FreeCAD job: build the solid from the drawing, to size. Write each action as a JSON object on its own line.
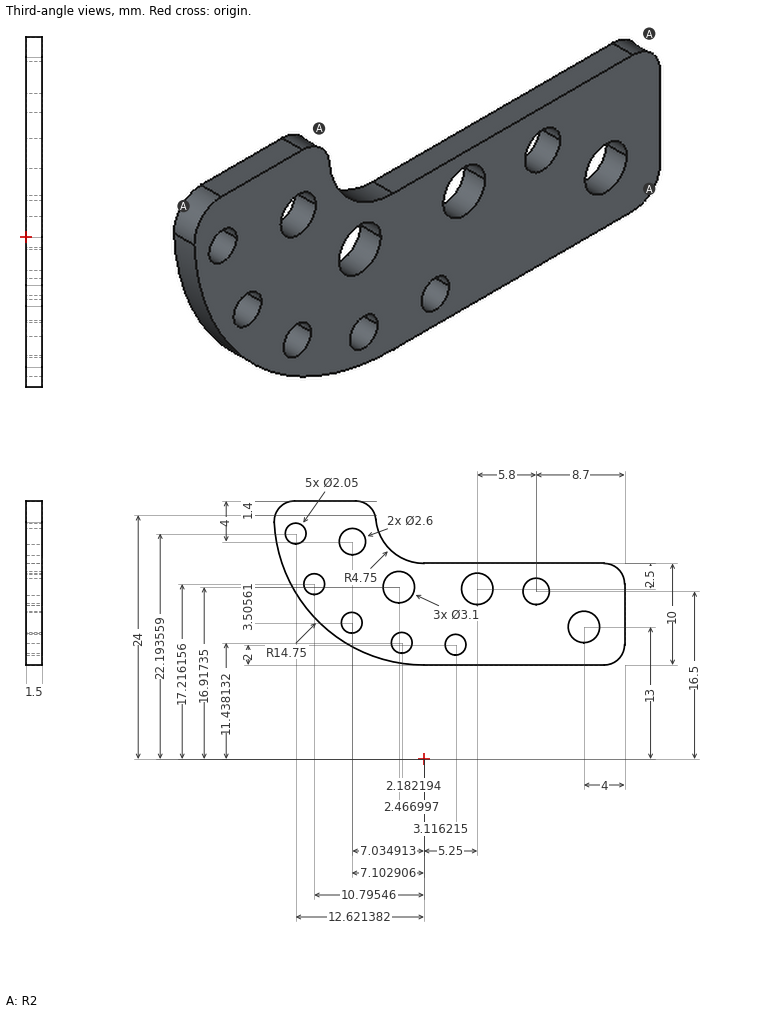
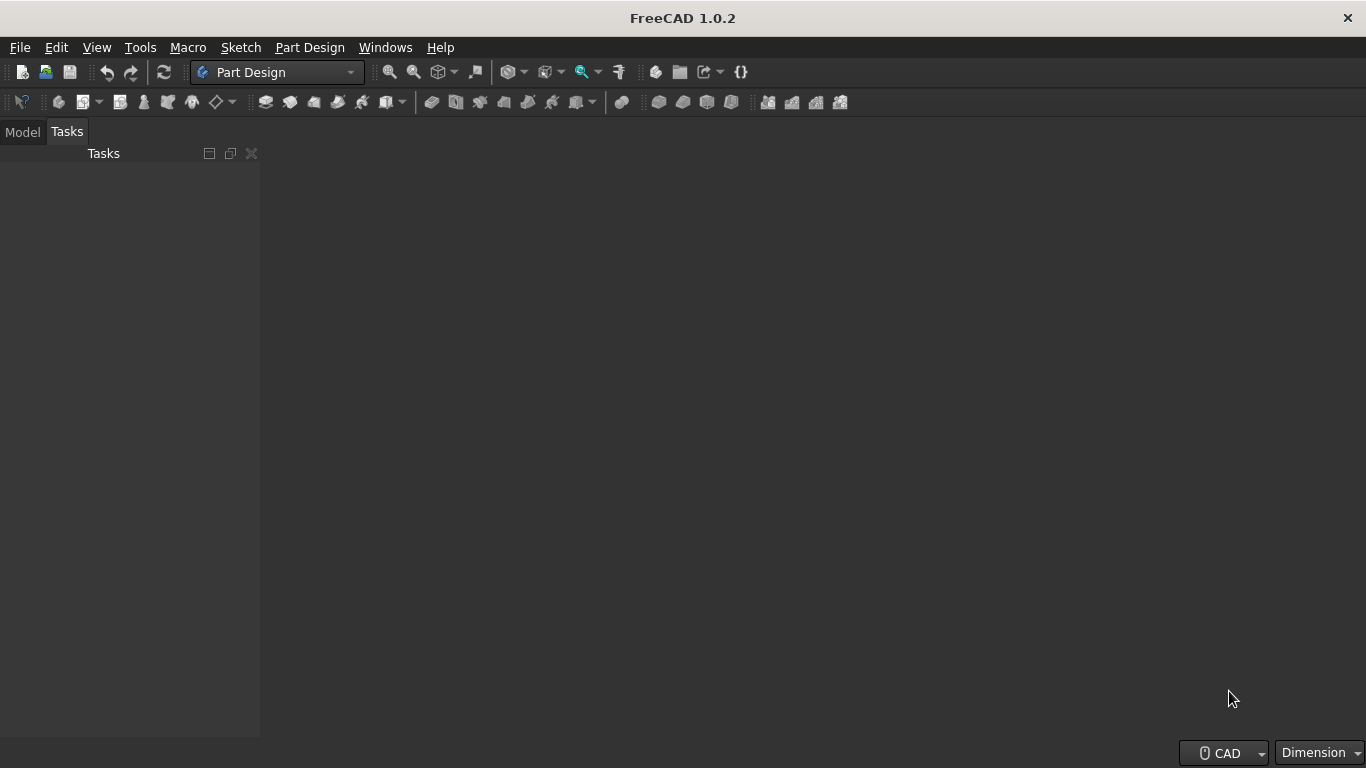
{"action": "left_click", "coordinate": [22, 72]}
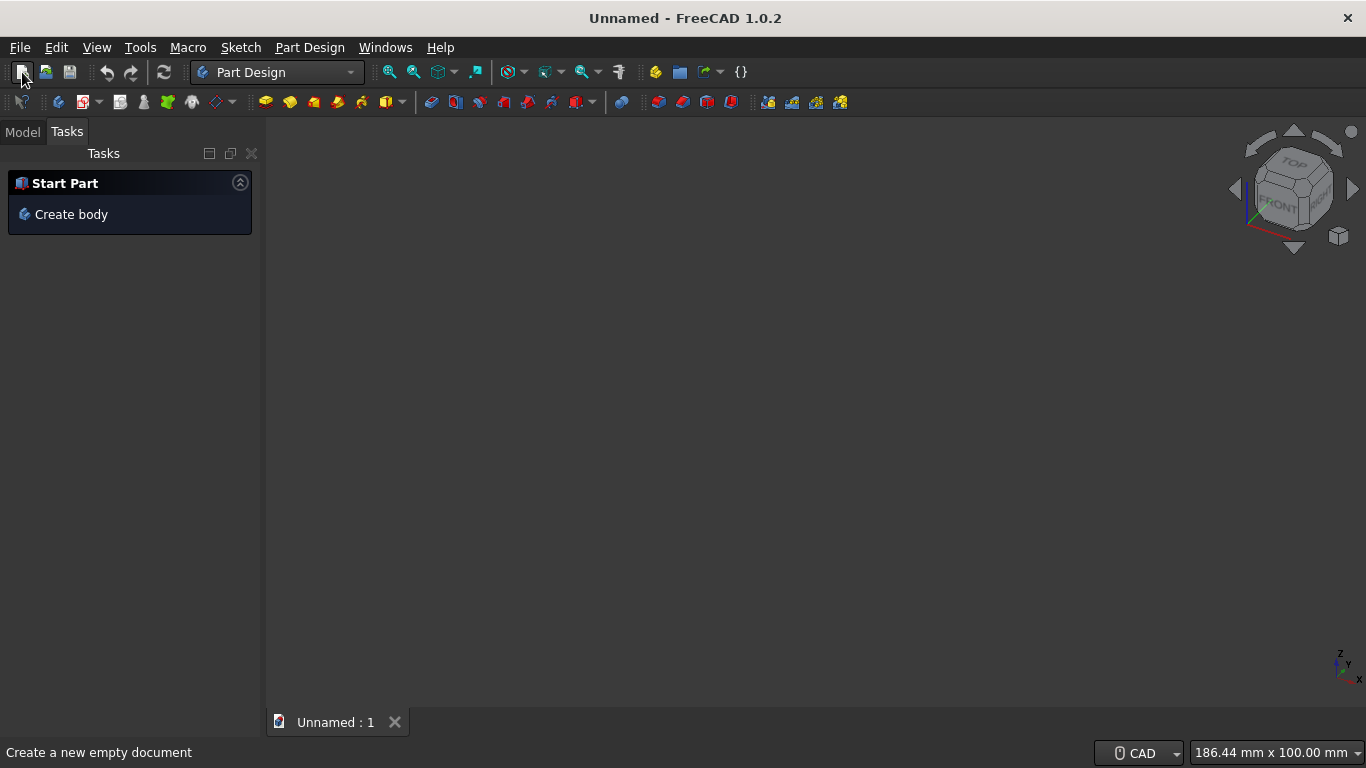
{"action": "left_click", "coordinate": [84, 102]}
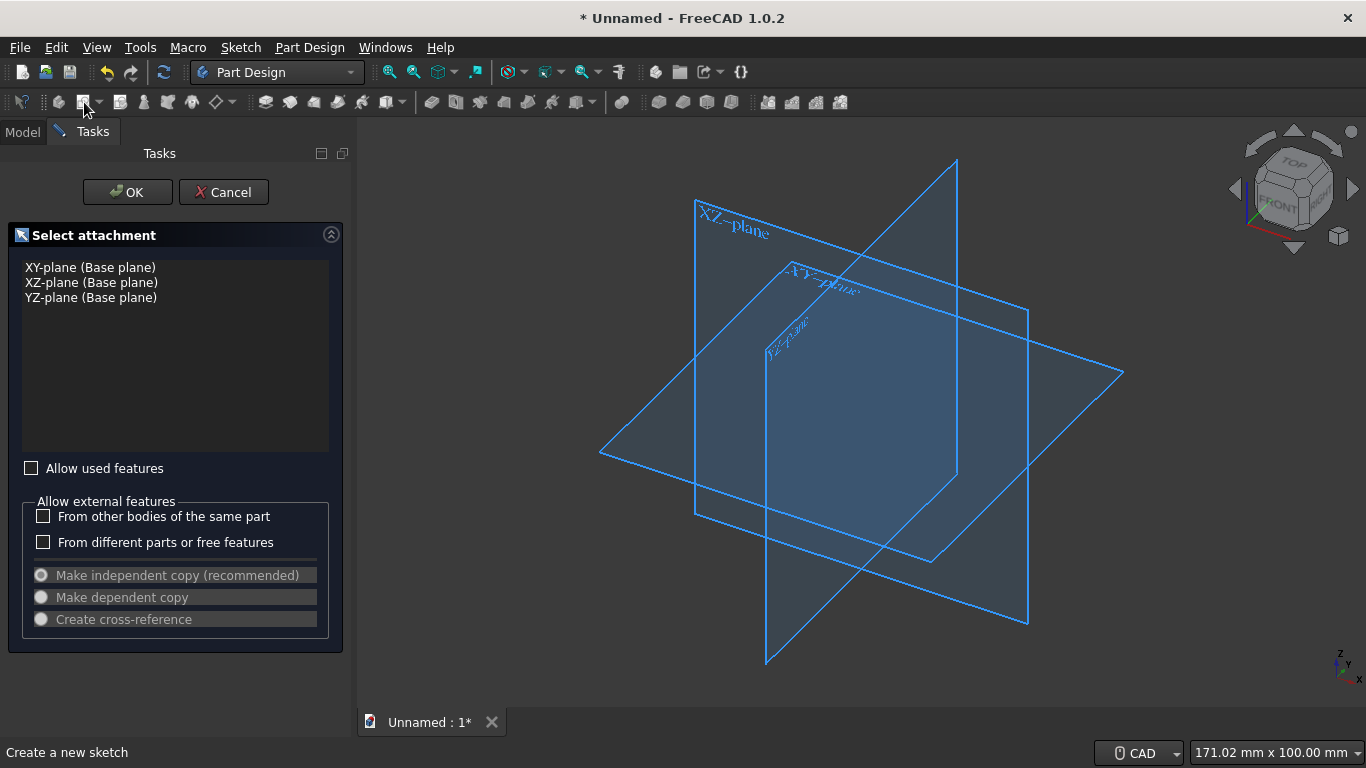
{"action": "left_click", "coordinate": [82, 298]}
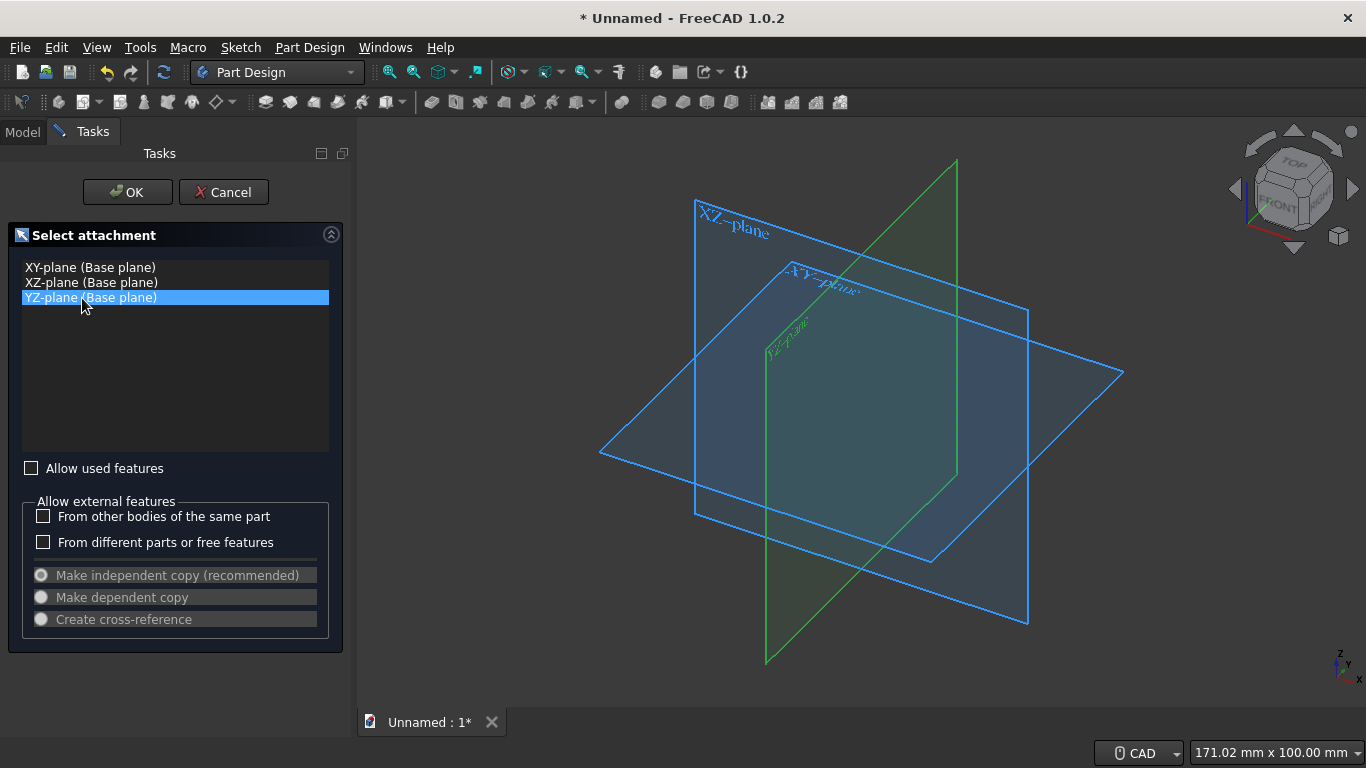
{"action": "left_click", "coordinate": [128, 192]}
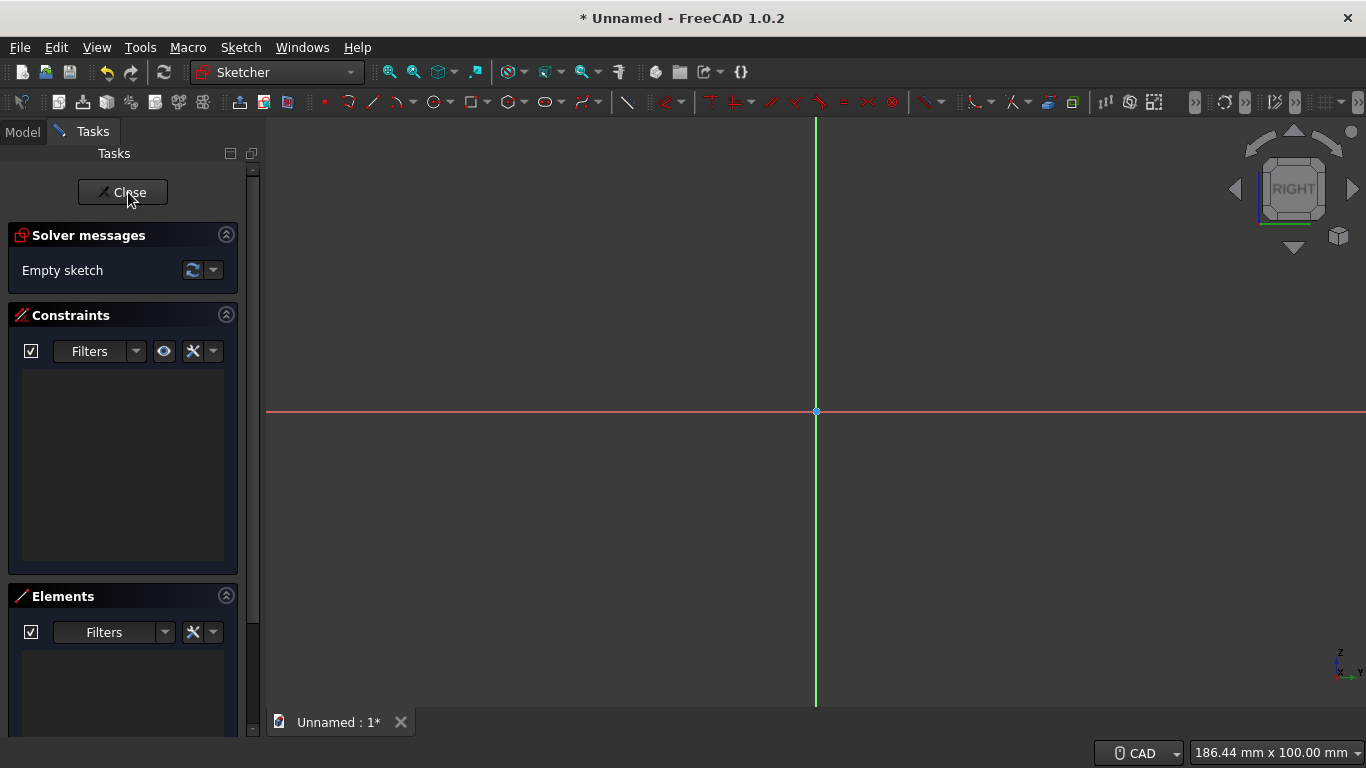
{"action": "scroll", "coordinate": [879, 293], "scroll_direction": "up", "scroll_amount": 5}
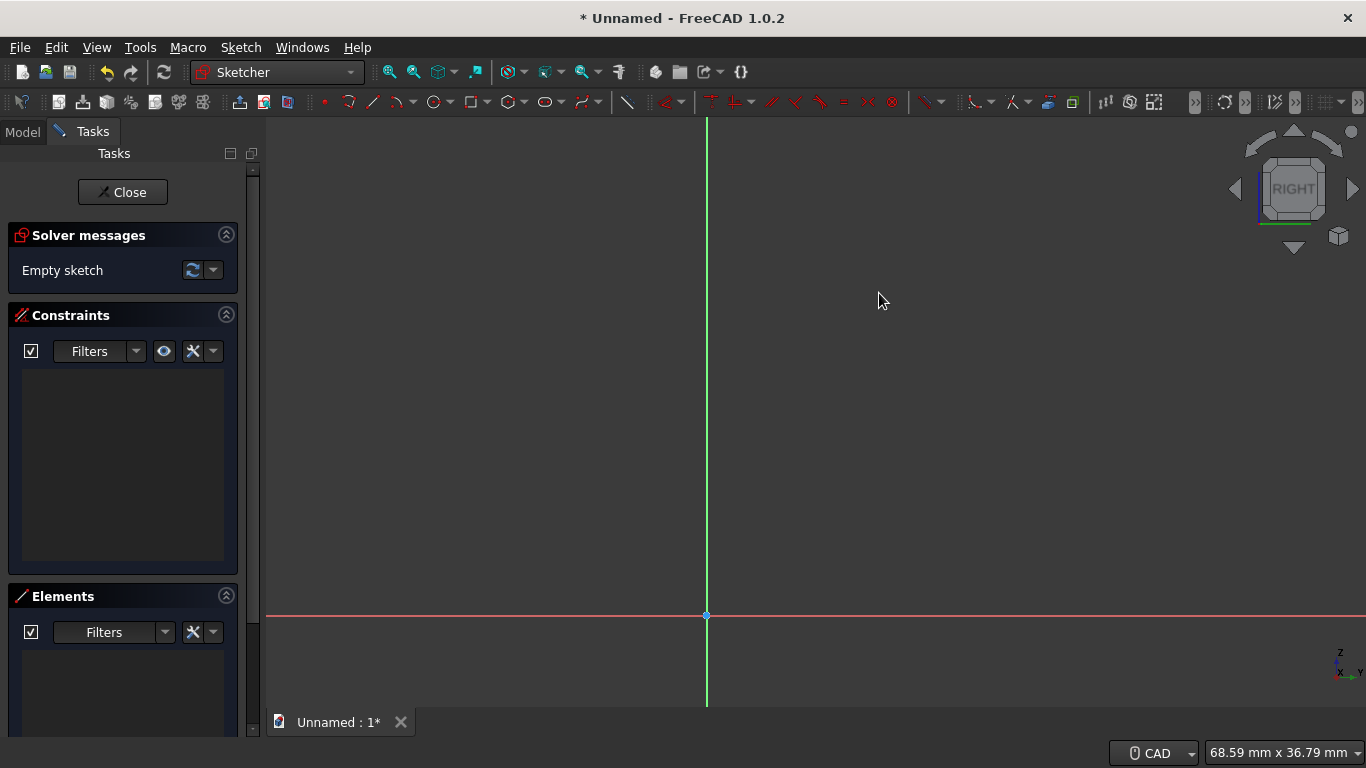
{"action": "left_click", "coordinate": [350, 102]}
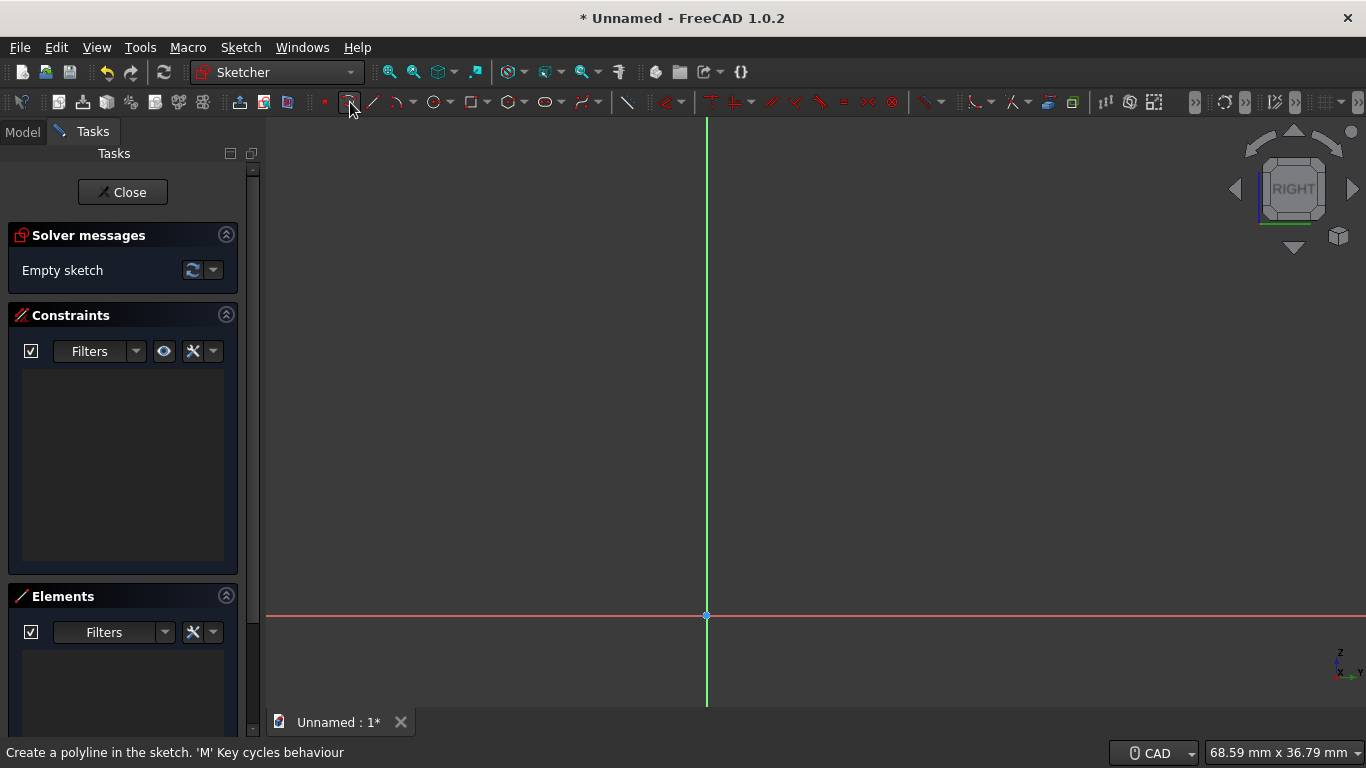
{"action": "left_click", "coordinate": [707, 468]}
{"action": "left_click", "coordinate": [1024, 468]}
{"action": "left_click", "coordinate": [1024, 307]}
{"action": "left_click", "coordinate": [707, 307]}
{"action": "right_click", "coordinate": [707, 307]}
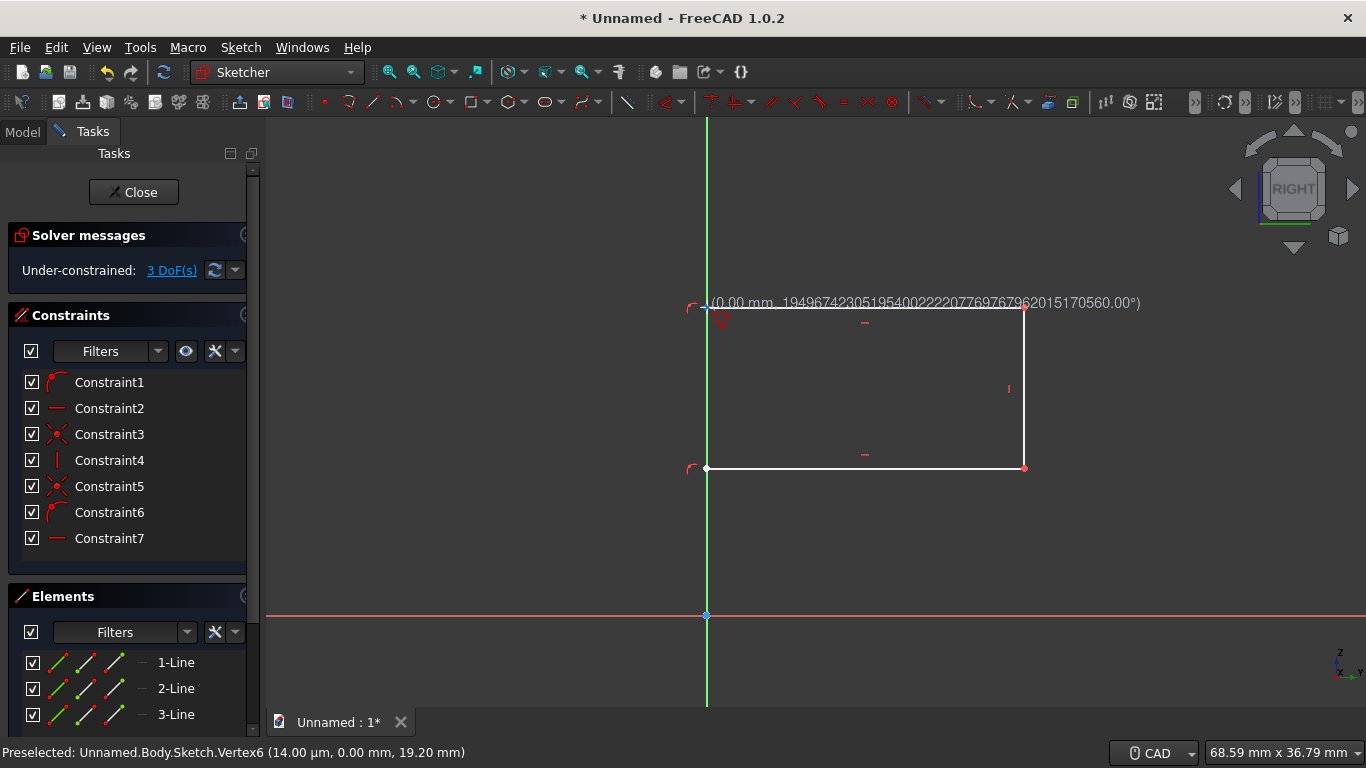
{"action": "left_click", "coordinate": [631, 231]}
{"action": "left_click", "coordinate": [631, 209]}
{"action": "left_click", "coordinate": [470, 209]}
{"action": "left_click", "coordinate": [470, 231]}
{"action": "right_click", "coordinate": [470, 231]}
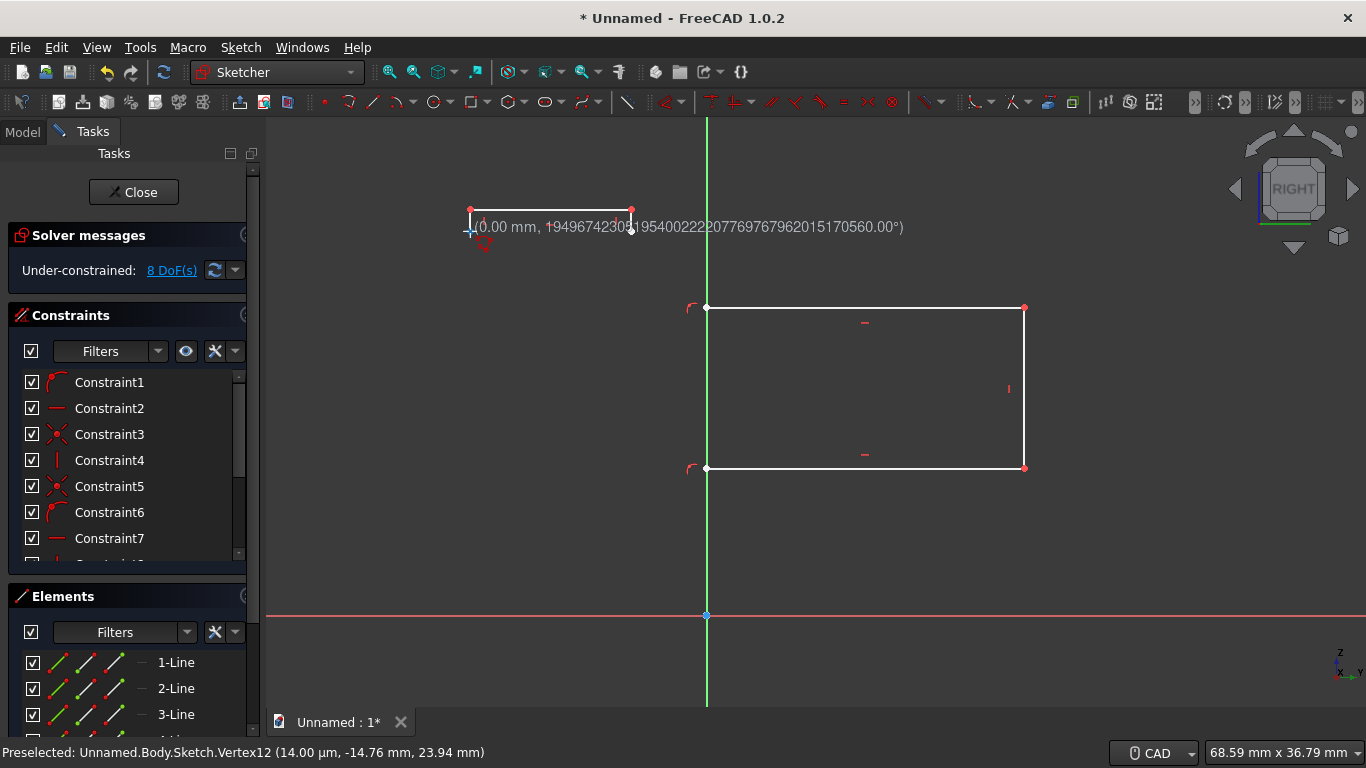
{"action": "key", "text": "g 3 a"}